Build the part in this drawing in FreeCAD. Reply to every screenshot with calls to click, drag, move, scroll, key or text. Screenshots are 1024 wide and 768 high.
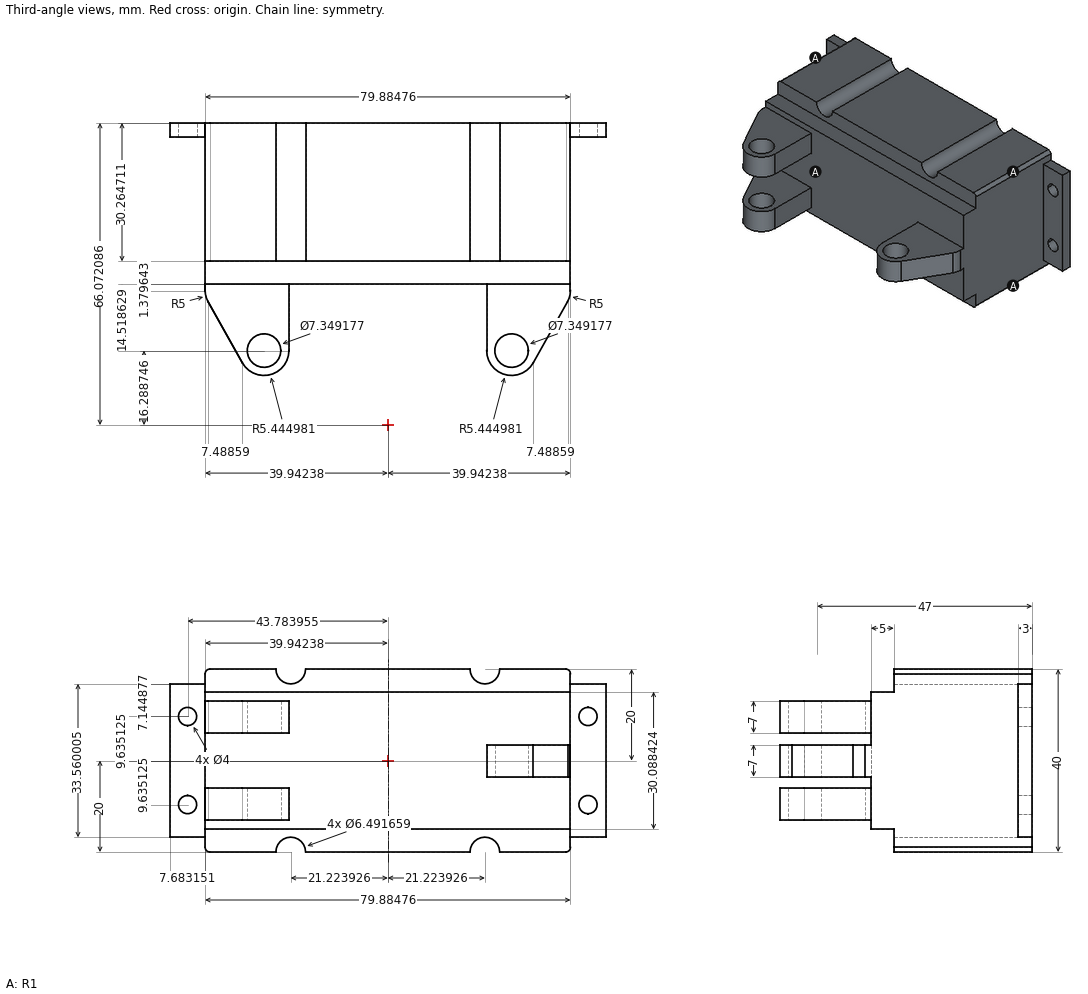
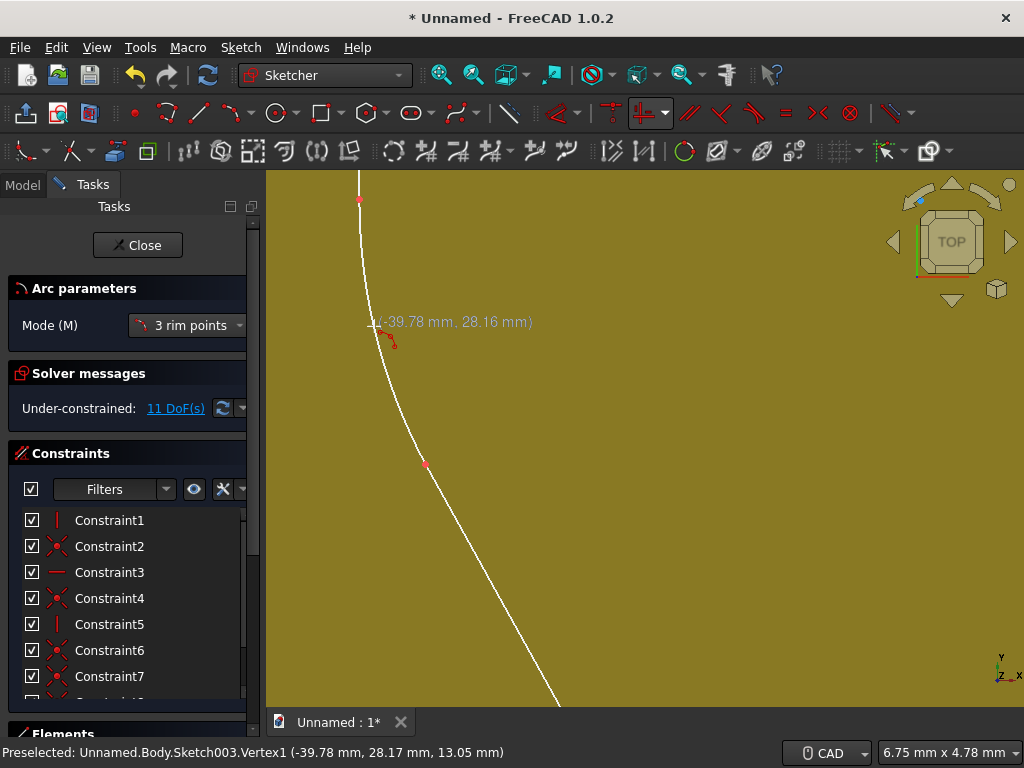
click(276, 114)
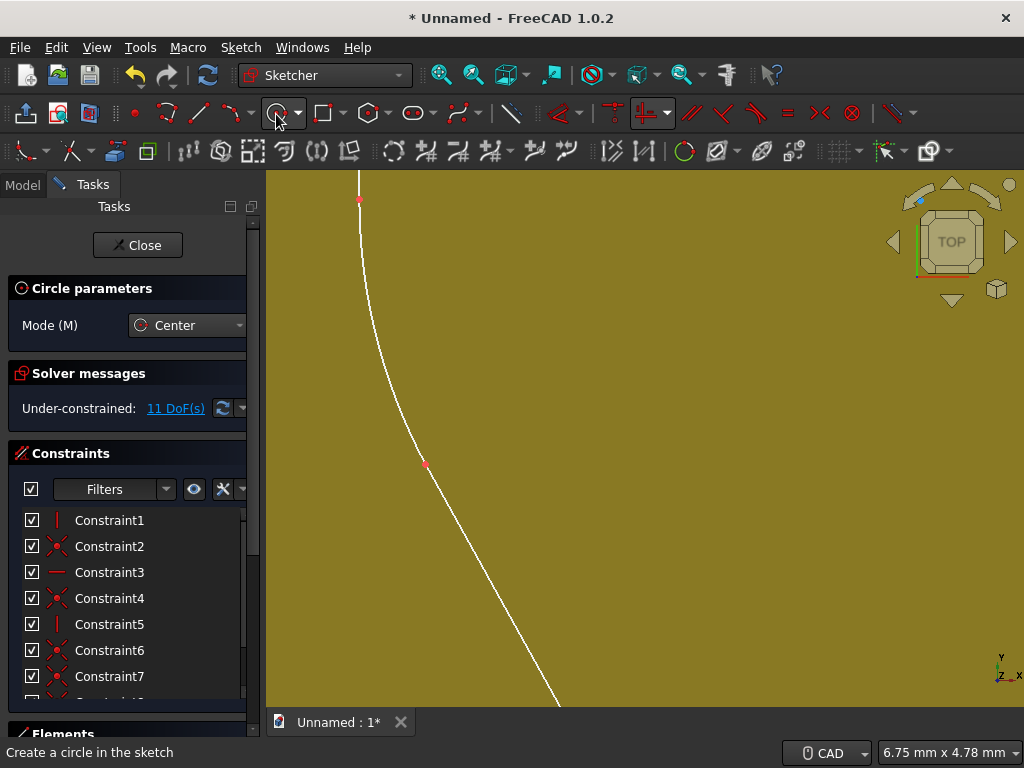
scroll(375, 307, down, 12)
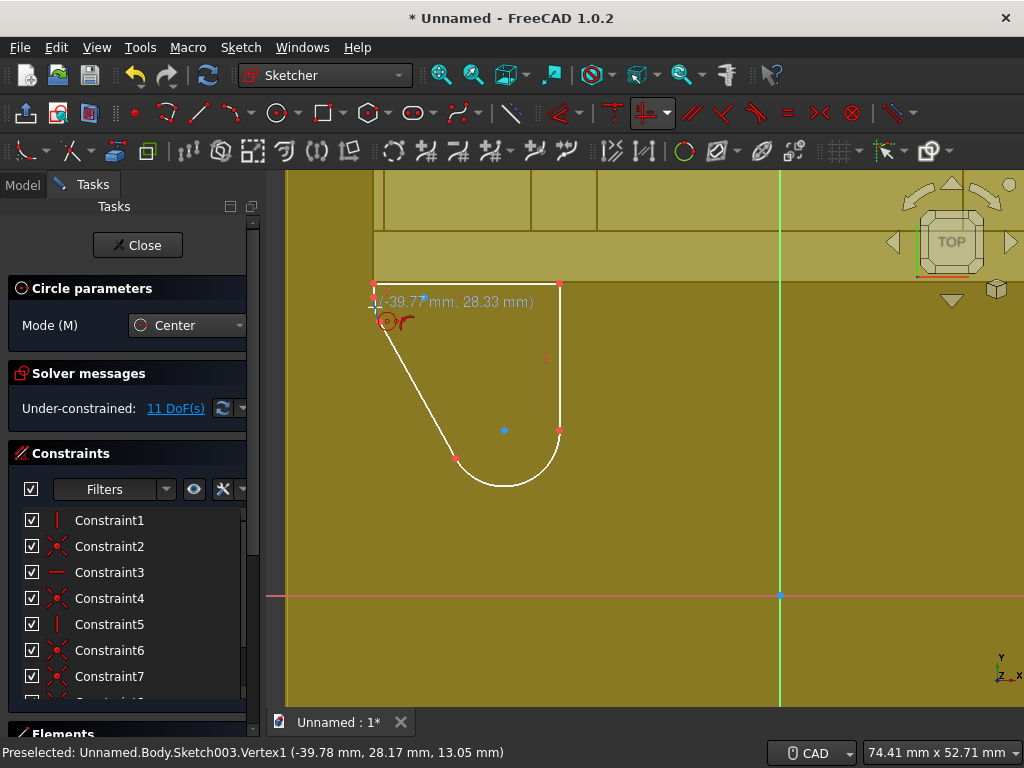
click(505, 430)
click(531, 403)
key(Escape)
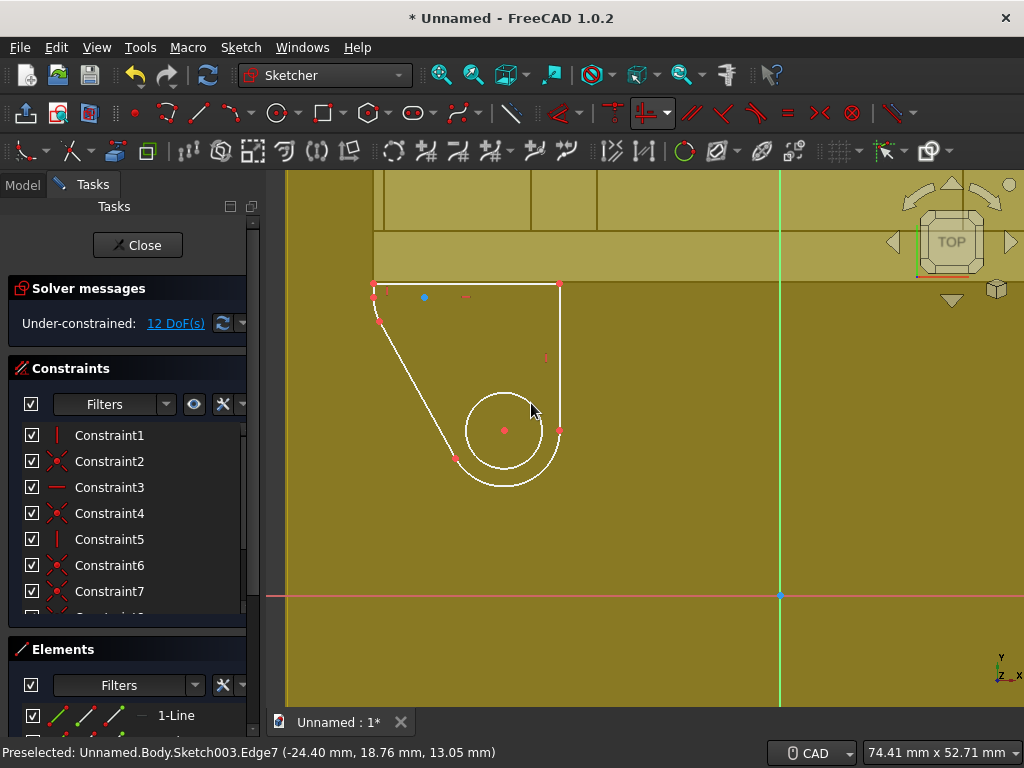
click(403, 363)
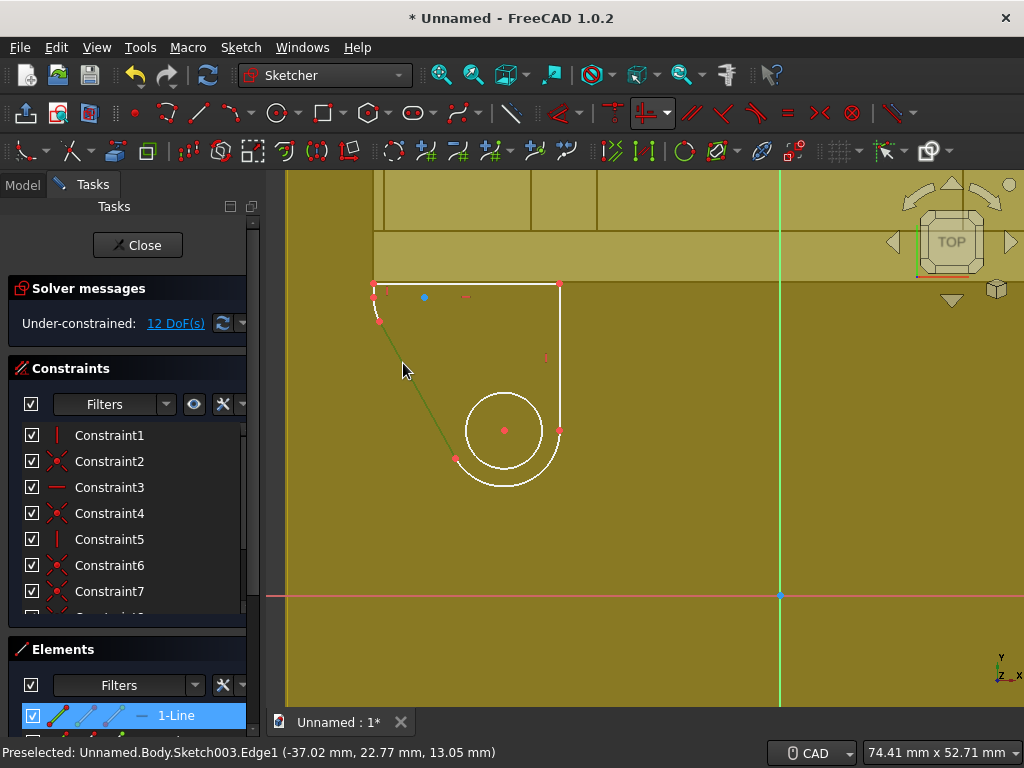
click(490, 485)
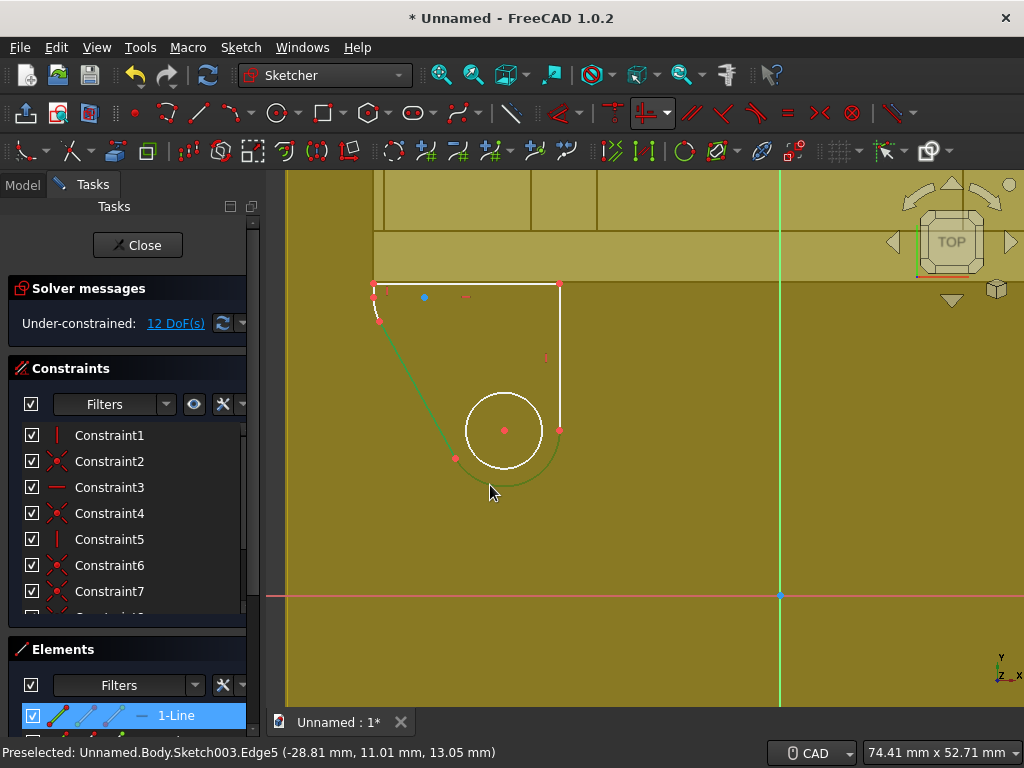
click(756, 114)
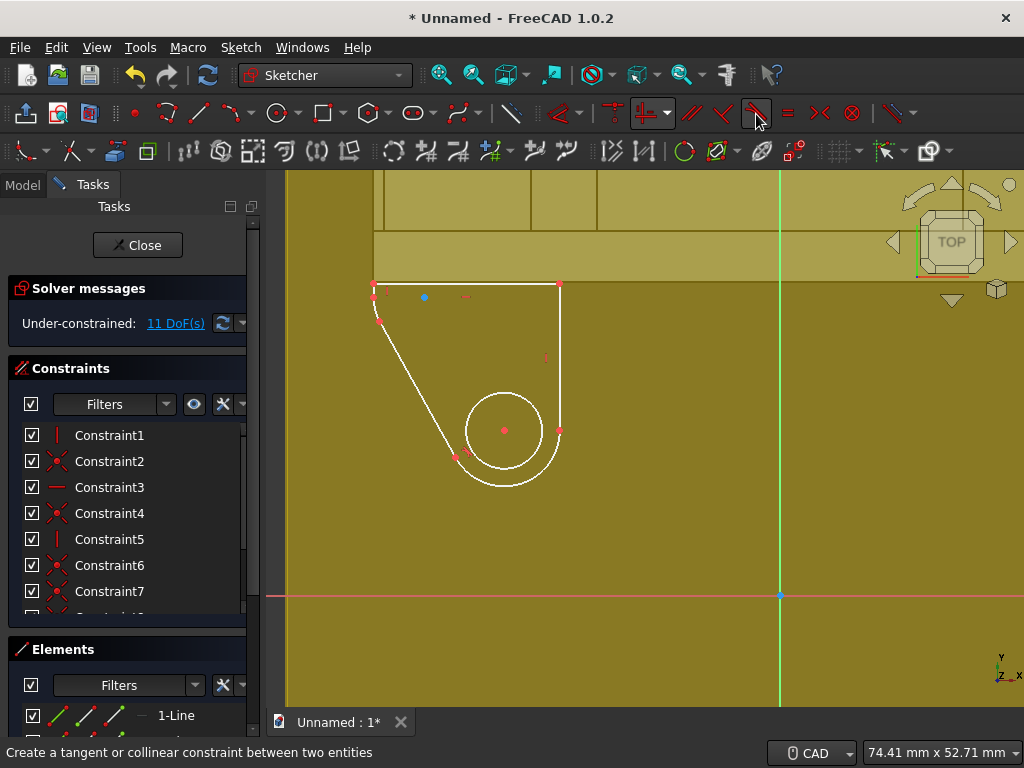
click(403, 362)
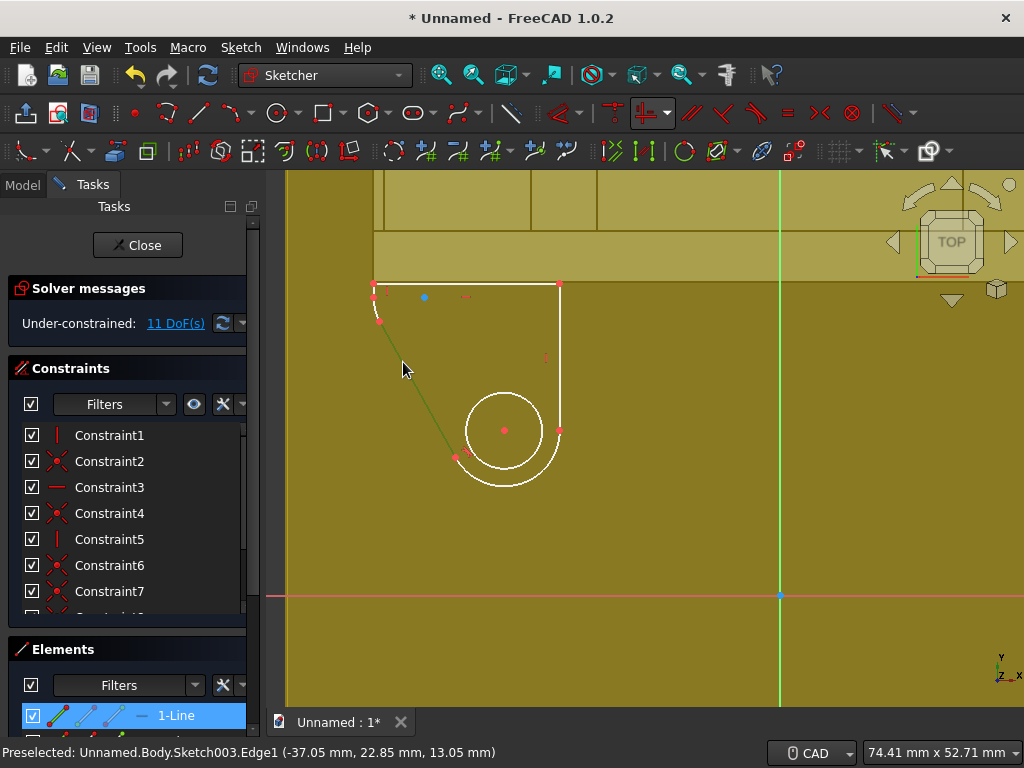
click(375, 310)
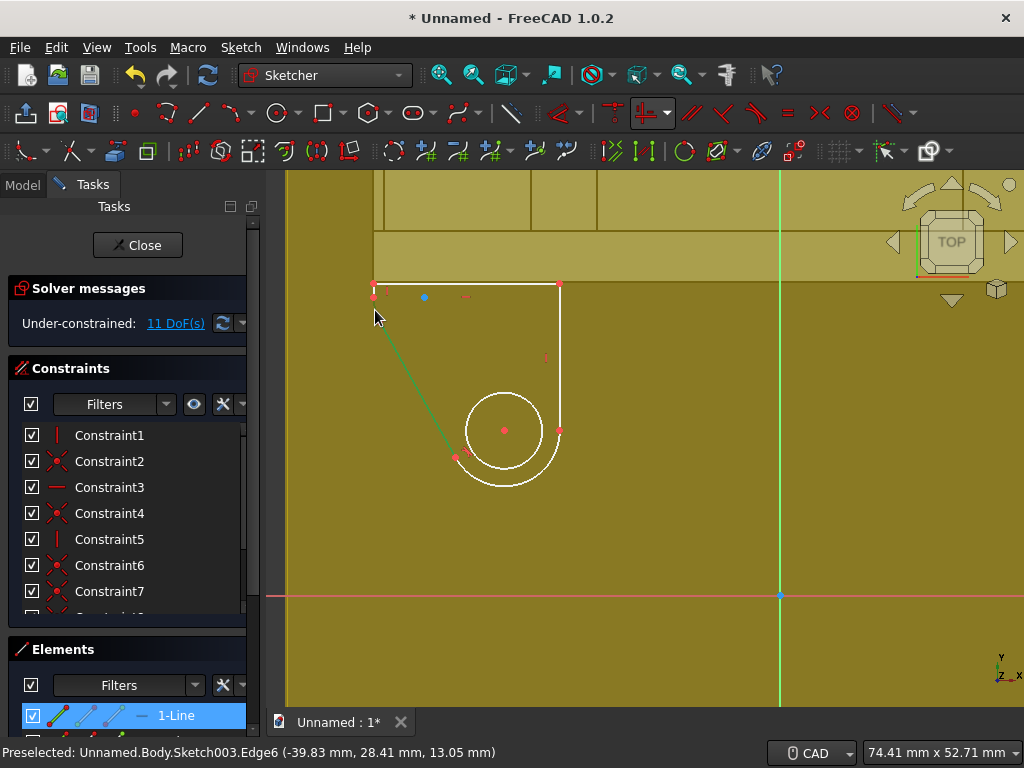
click(756, 114)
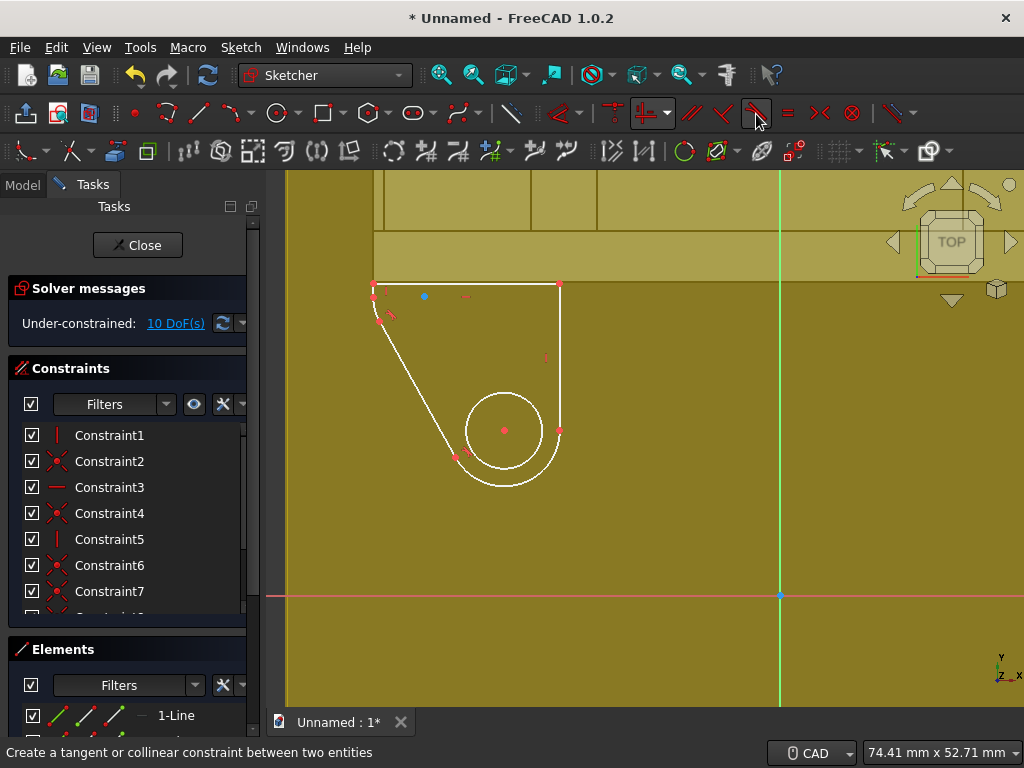
click(560, 386)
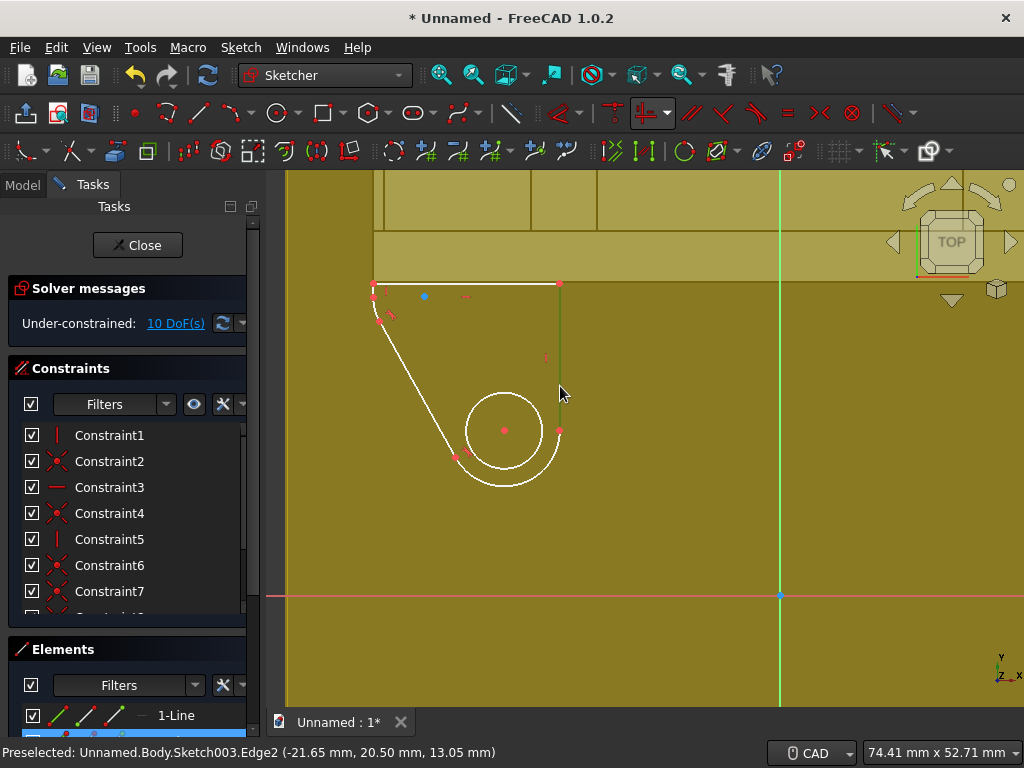
click(489, 484)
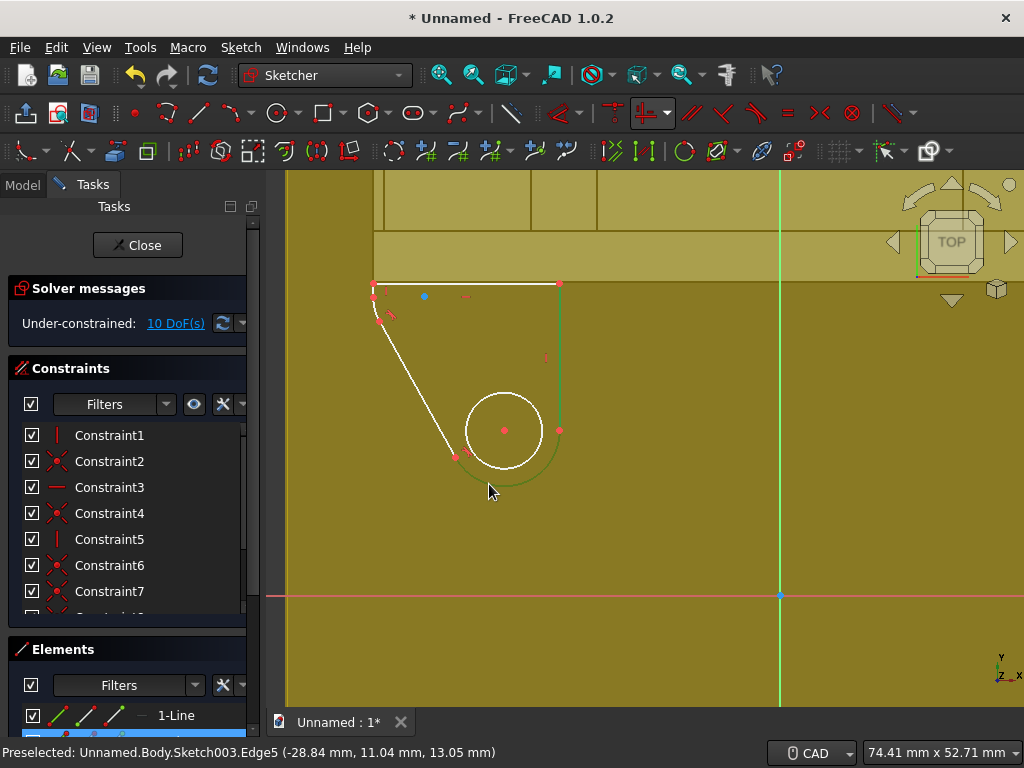
click(756, 114)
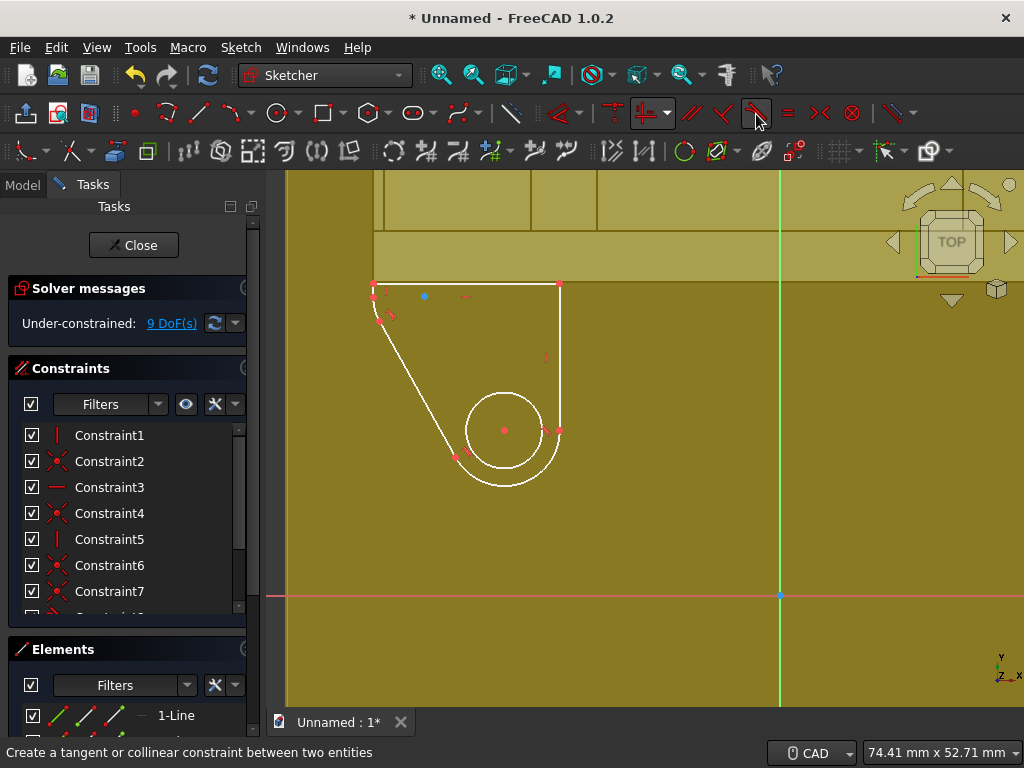
scroll(373, 291, up, 4)